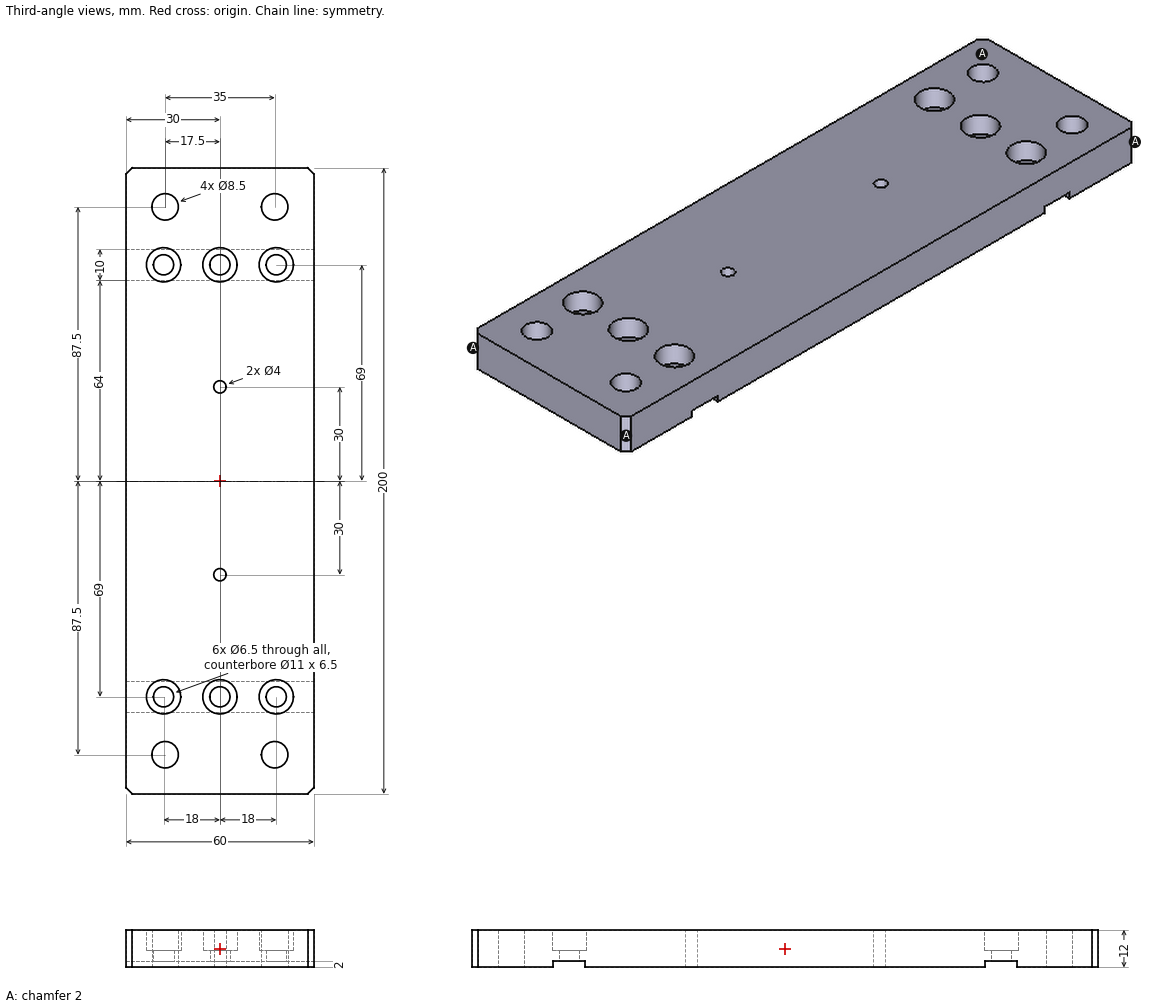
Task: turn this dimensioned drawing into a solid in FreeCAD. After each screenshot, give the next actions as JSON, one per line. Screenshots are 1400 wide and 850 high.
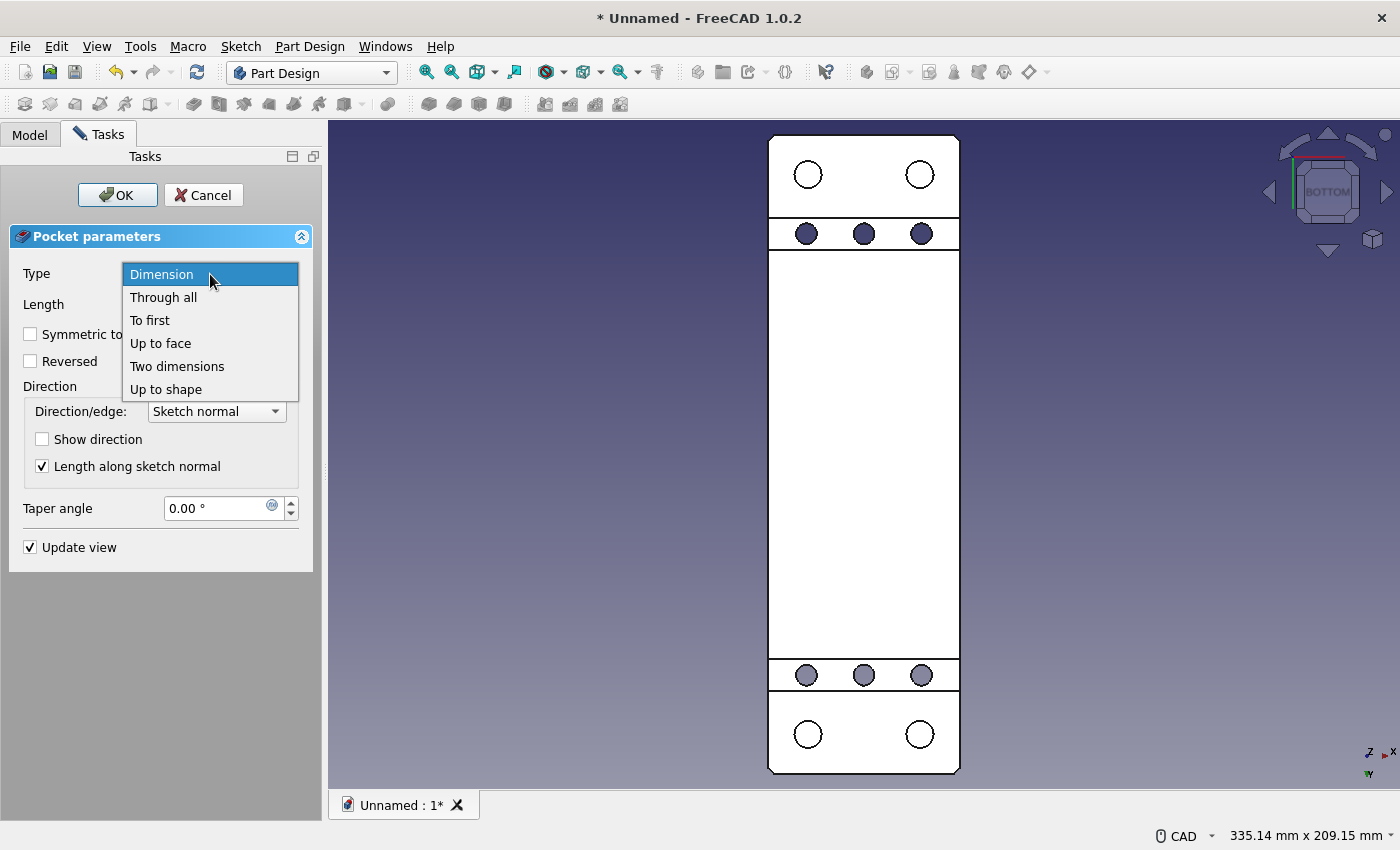
{"action": "left_click", "coordinate": [208, 298]}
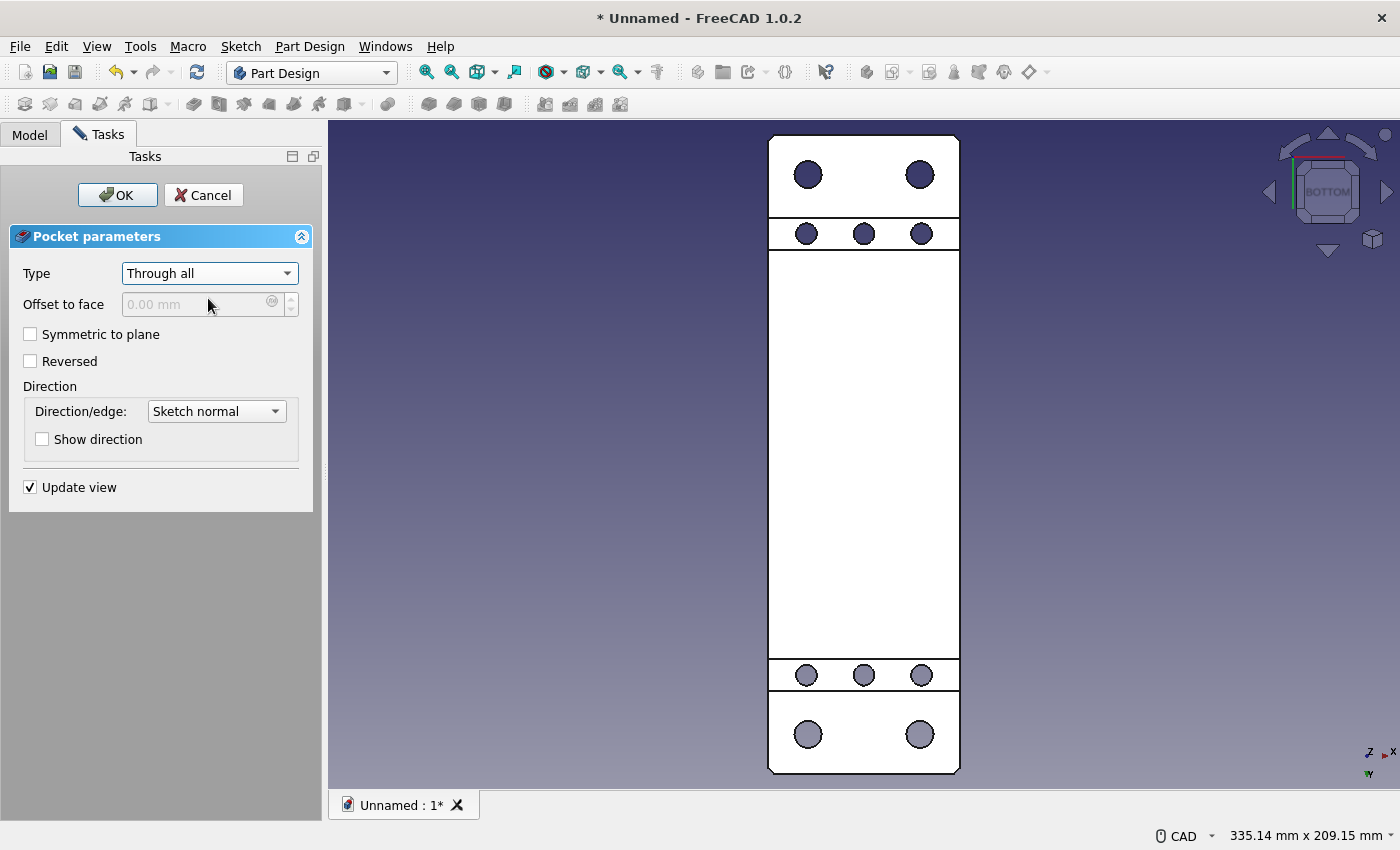
{"action": "left_click", "coordinate": [118, 195]}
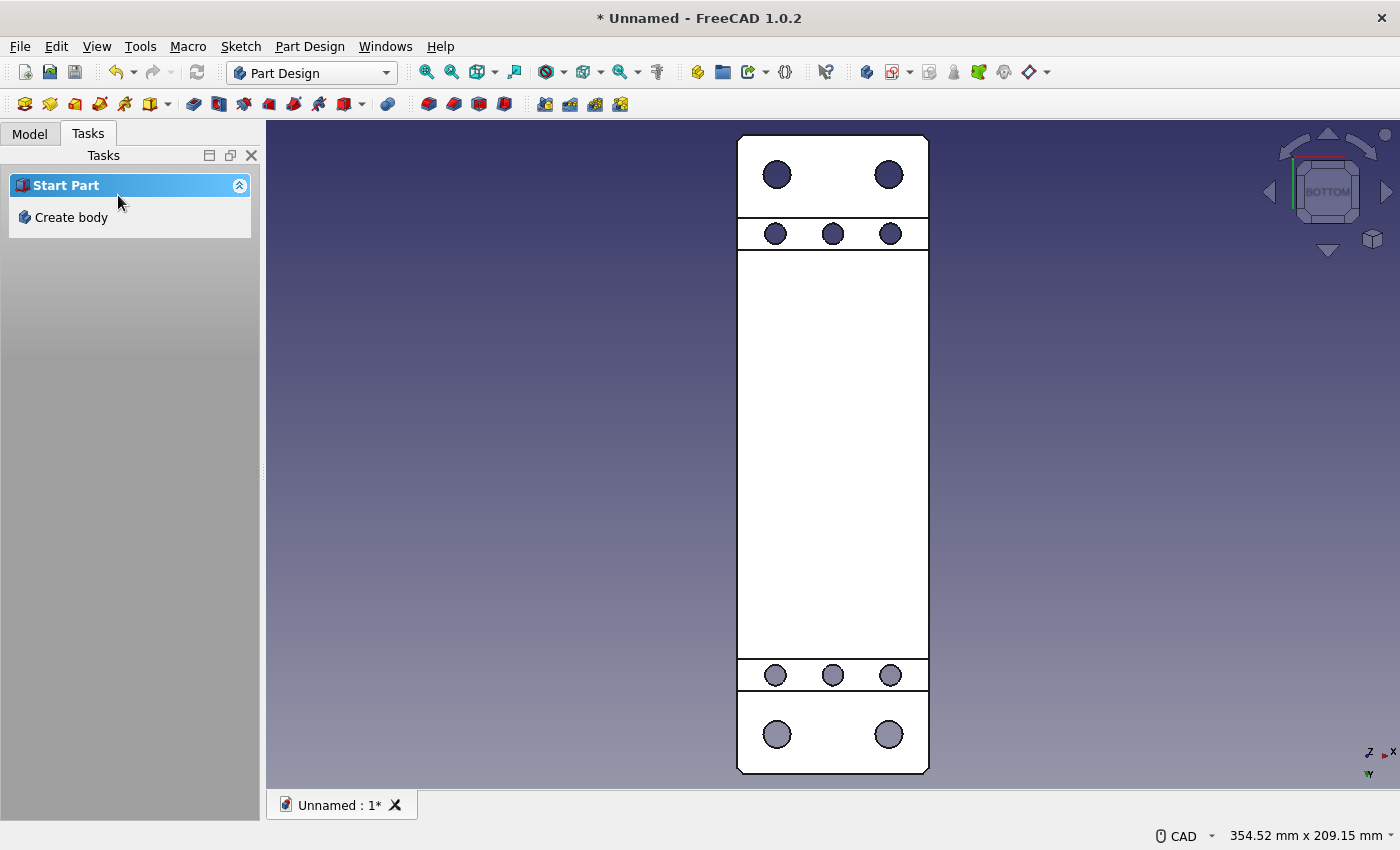
{"action": "key", "text": "0"}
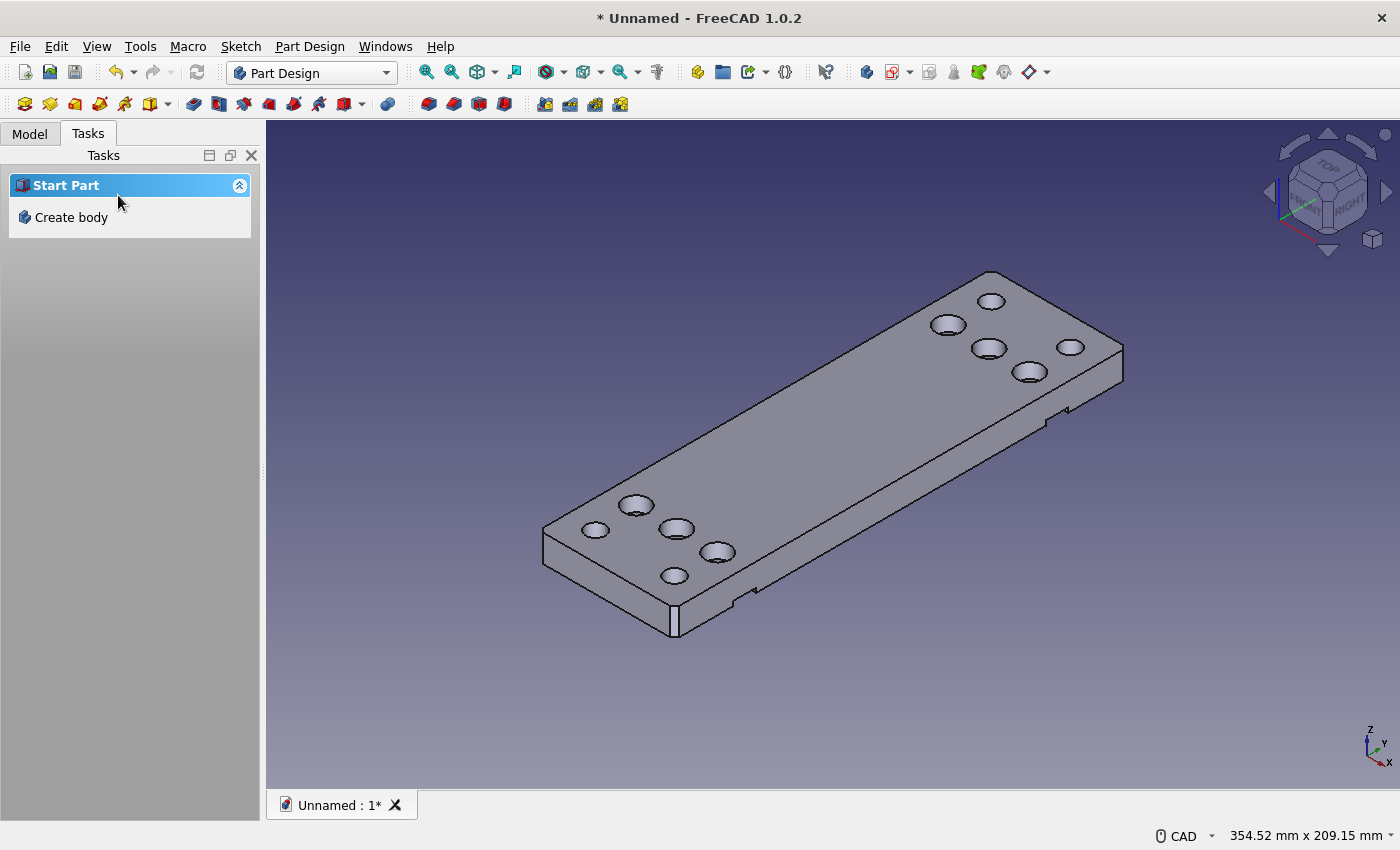
{"action": "left_click", "coordinate": [898, 401]}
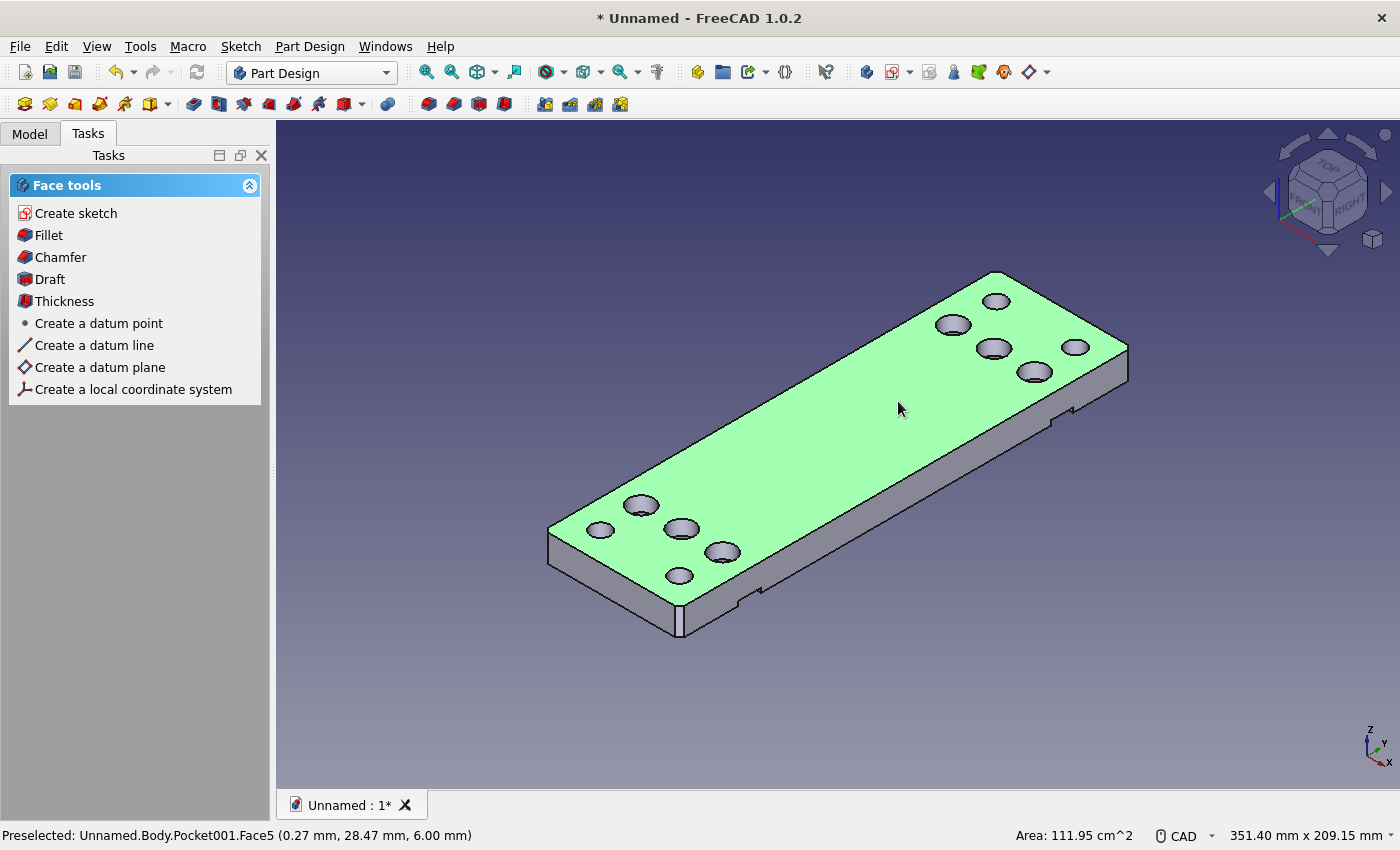
{"action": "left_click", "coordinate": [892, 72]}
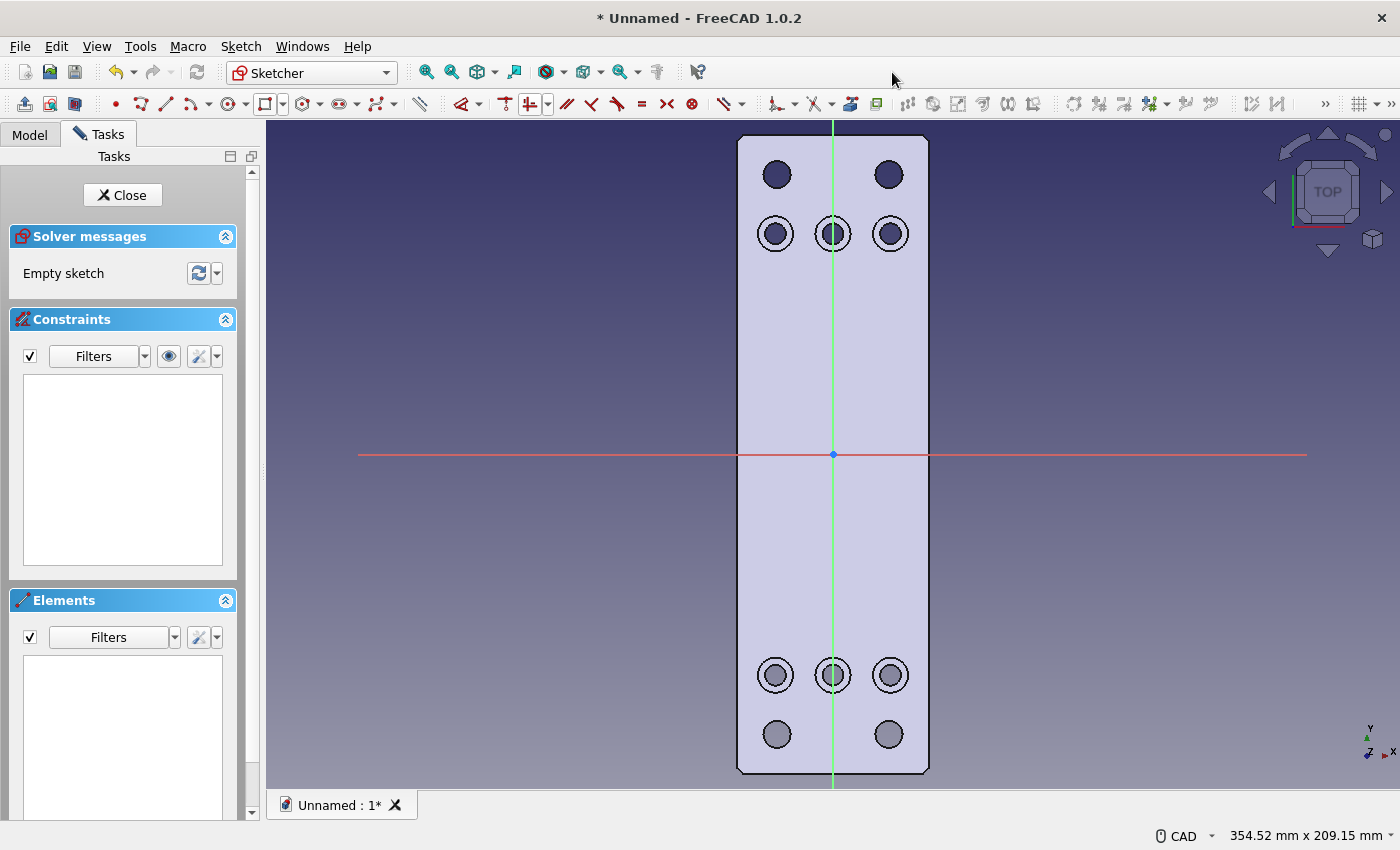
{"action": "scroll", "coordinate": [889, 454], "scroll_direction": "up", "scroll_amount": 4}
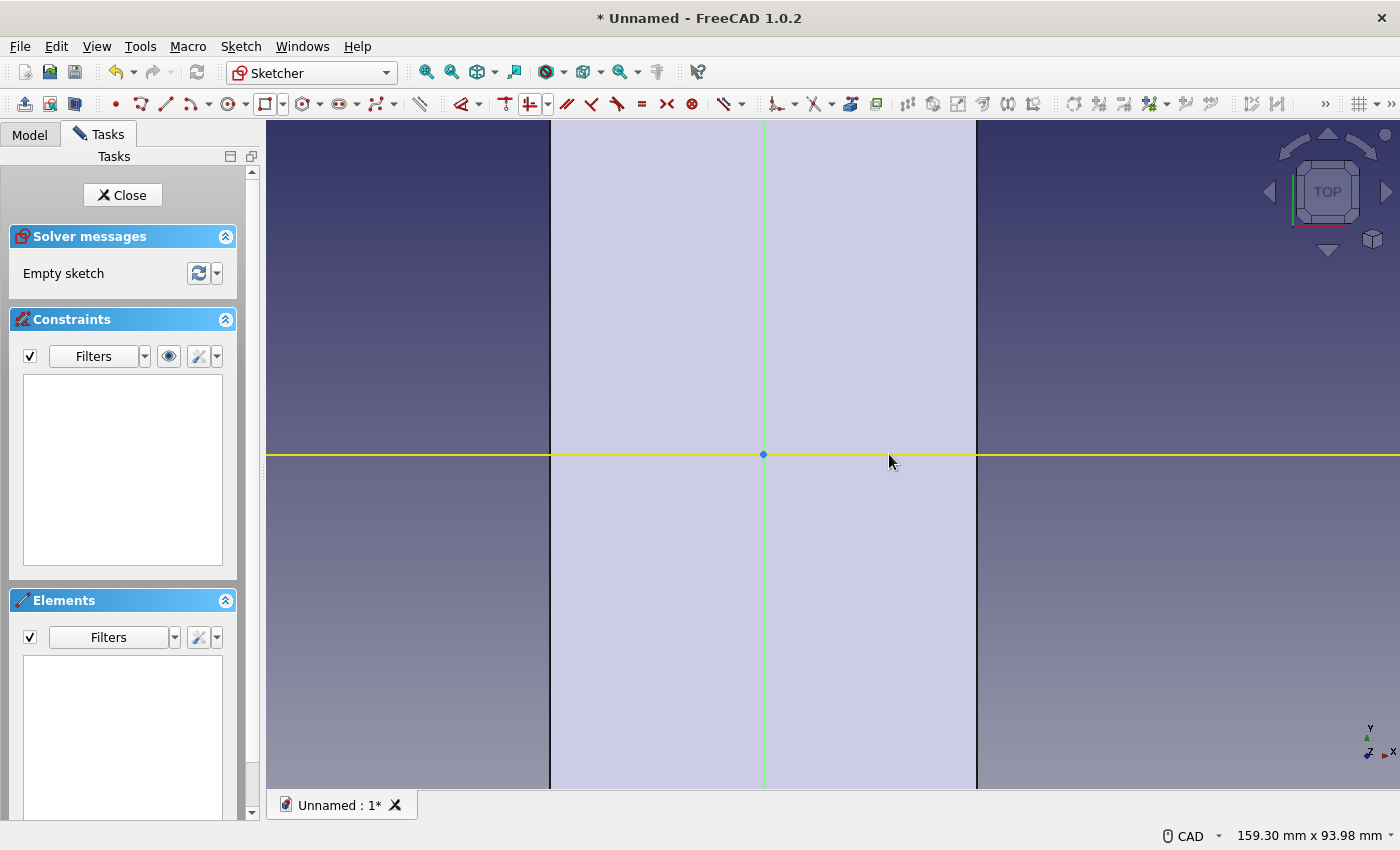
{"action": "left_click", "coordinate": [228, 104]}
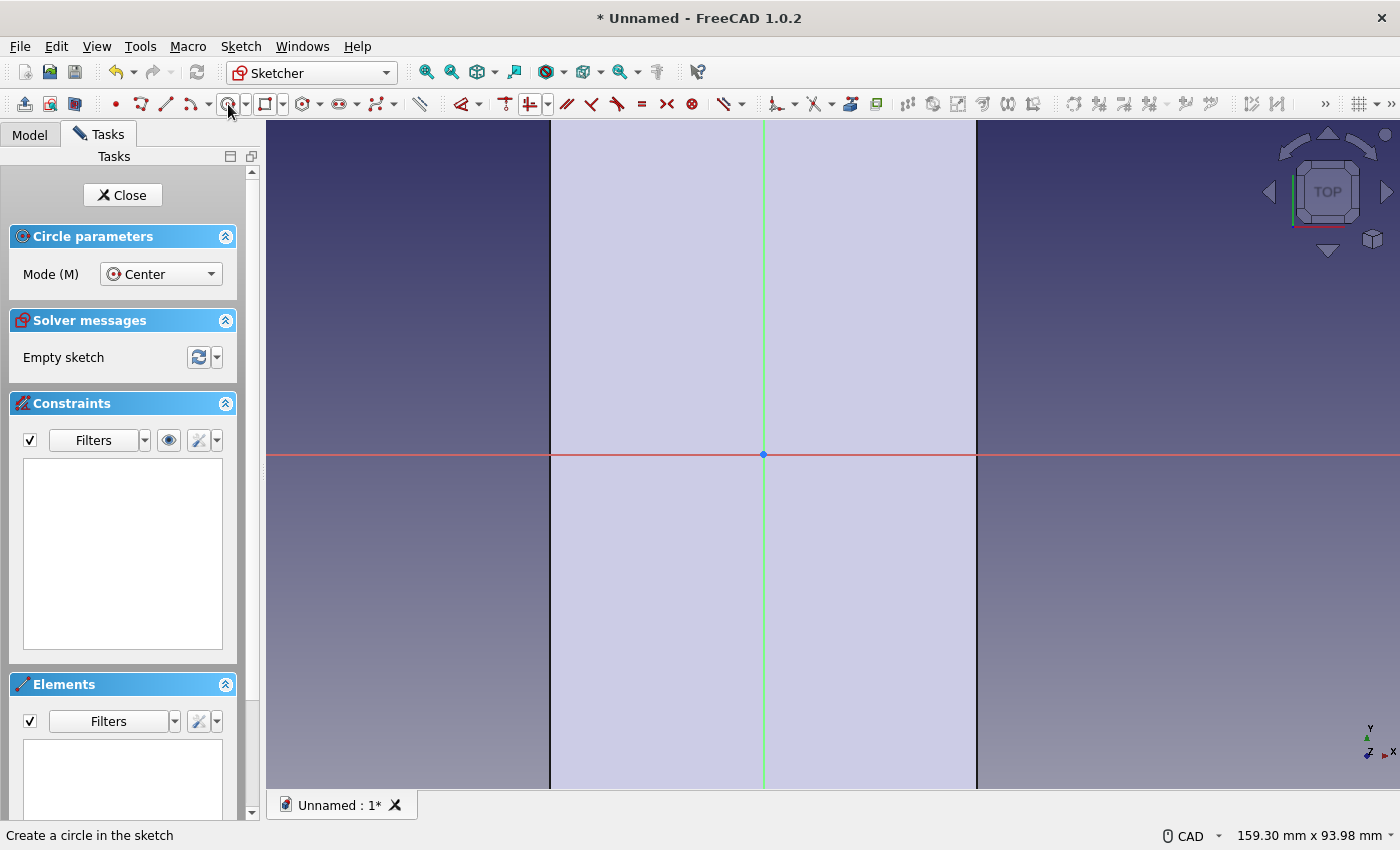
{"action": "scroll", "coordinate": [764, 241], "scroll_direction": "up", "scroll_amount": 3}